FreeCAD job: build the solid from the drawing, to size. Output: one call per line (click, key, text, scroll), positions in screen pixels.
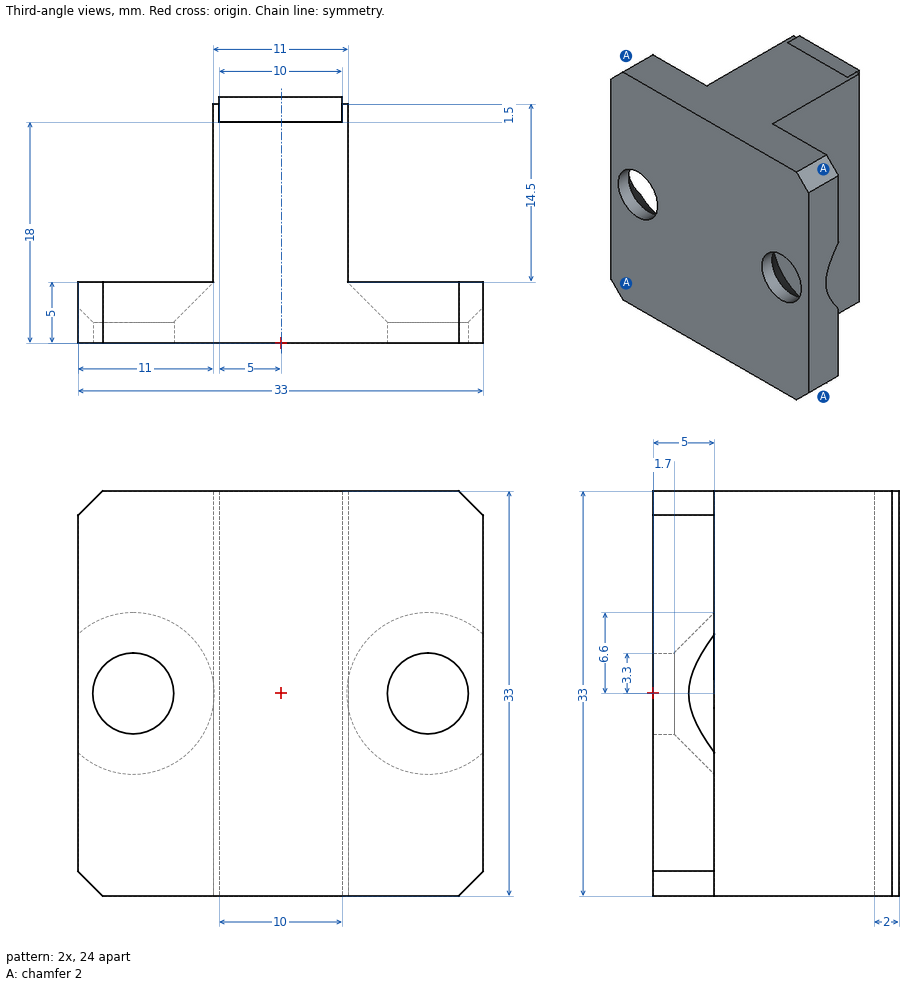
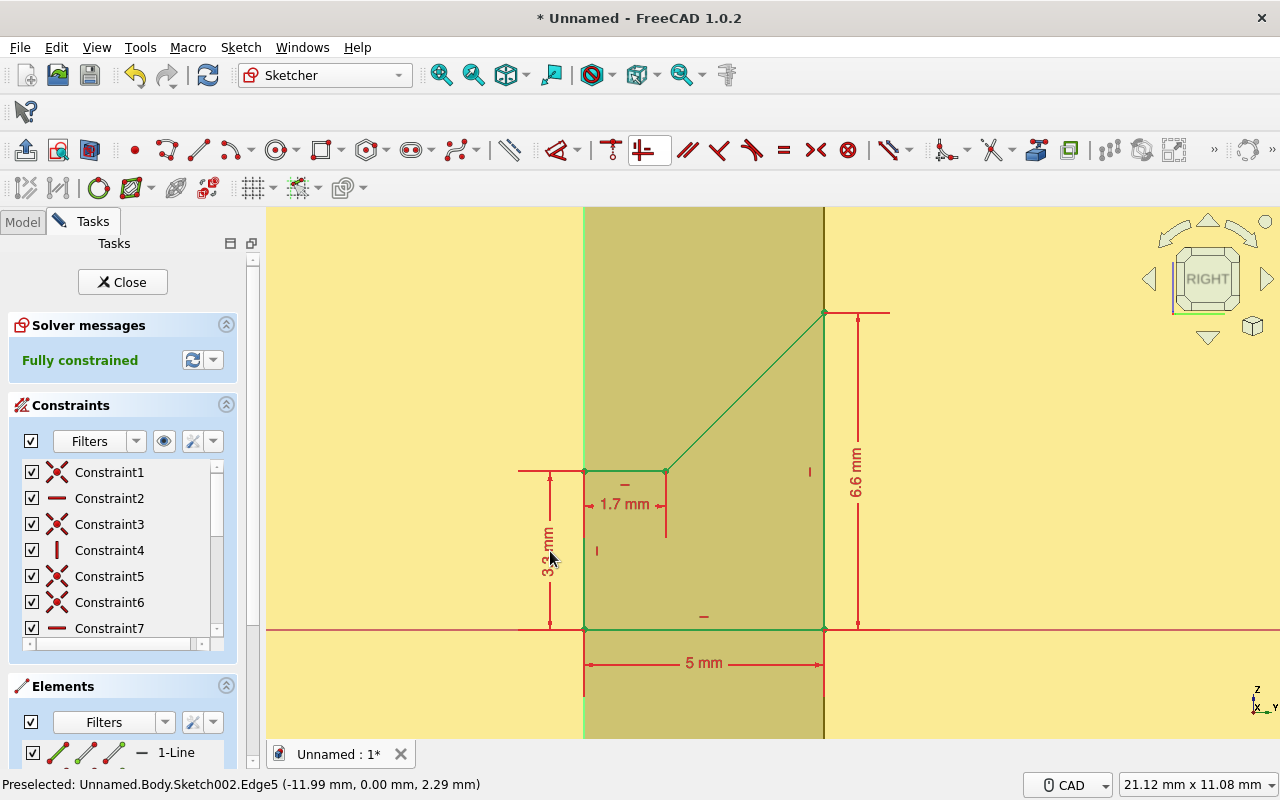
click(123, 282)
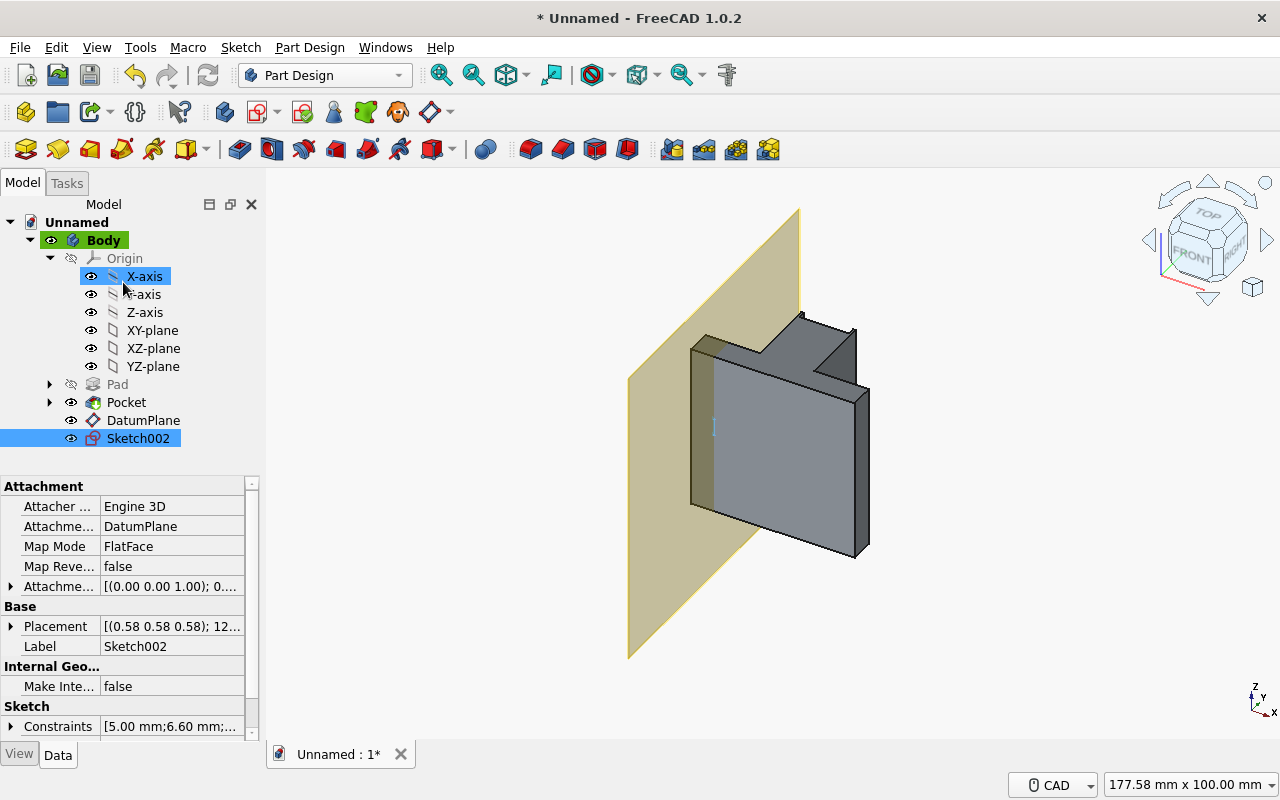
click(304, 150)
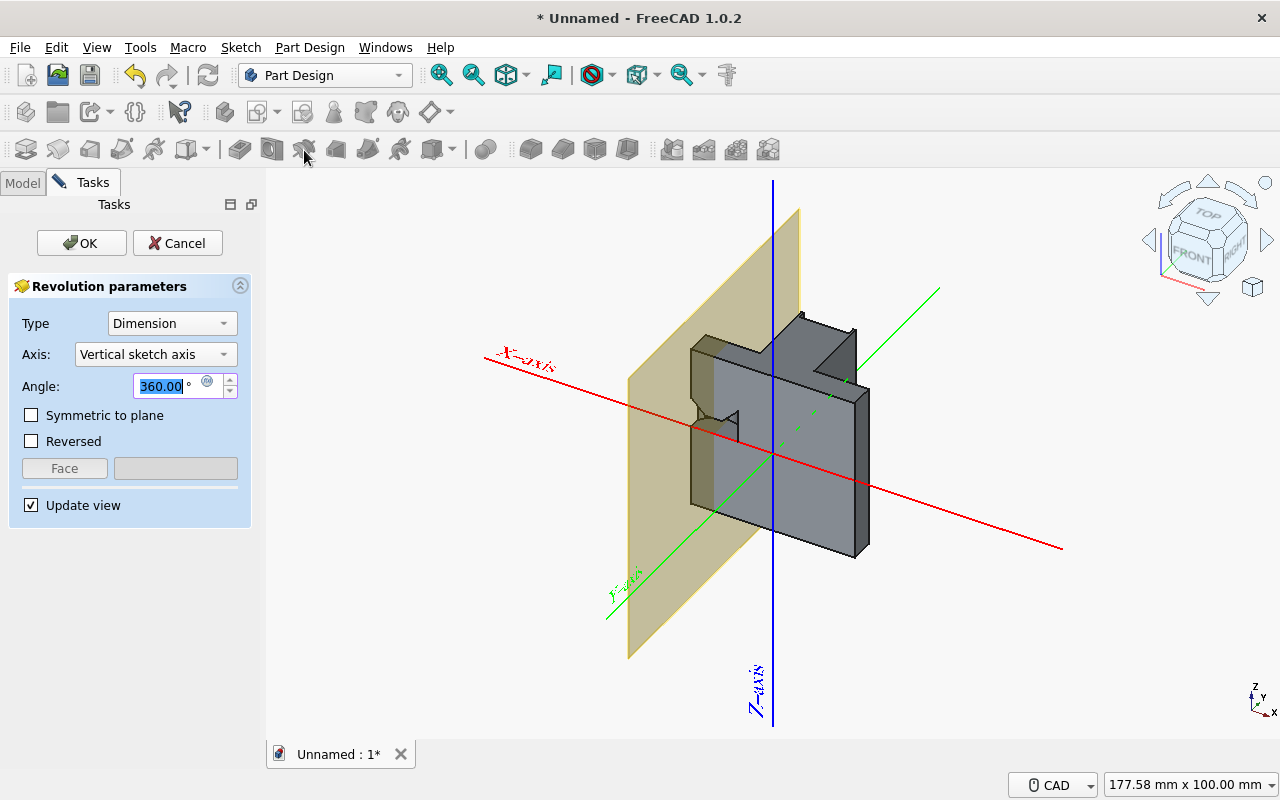
click(156, 354)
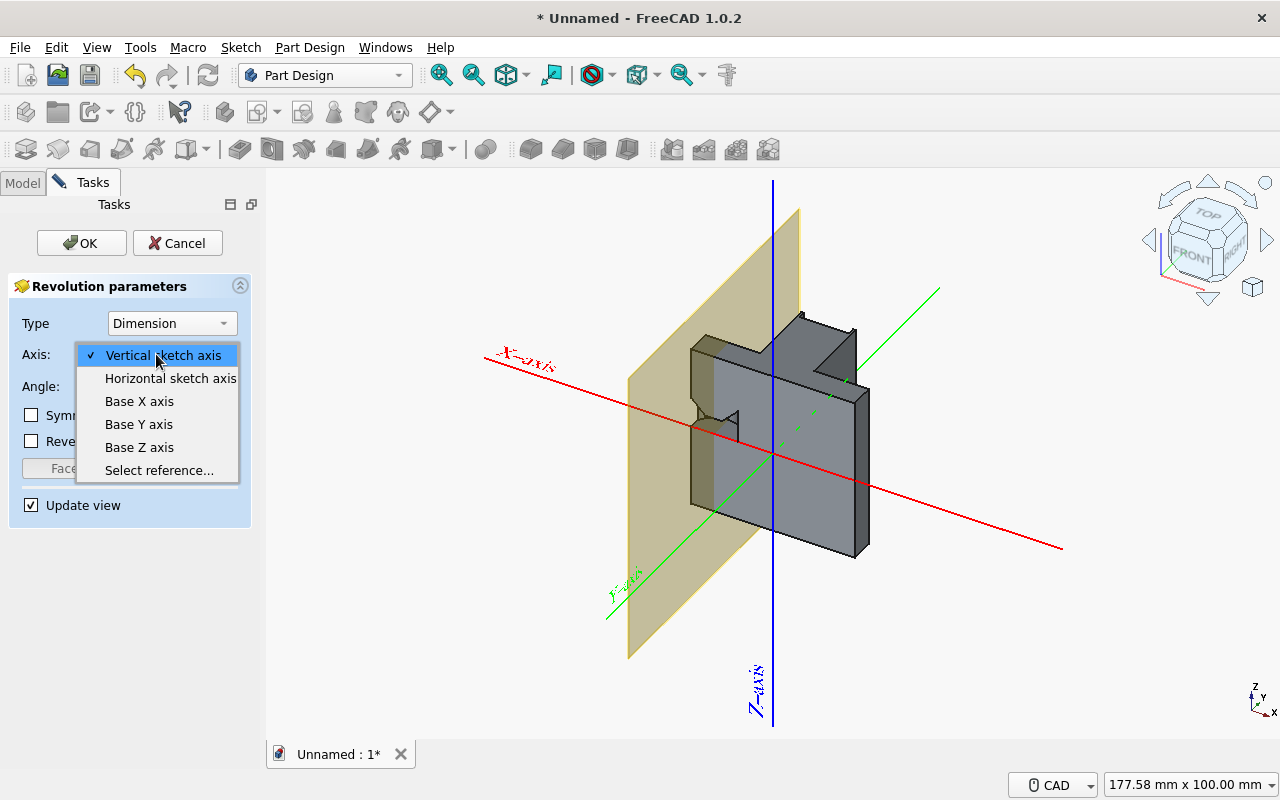
click(156, 378)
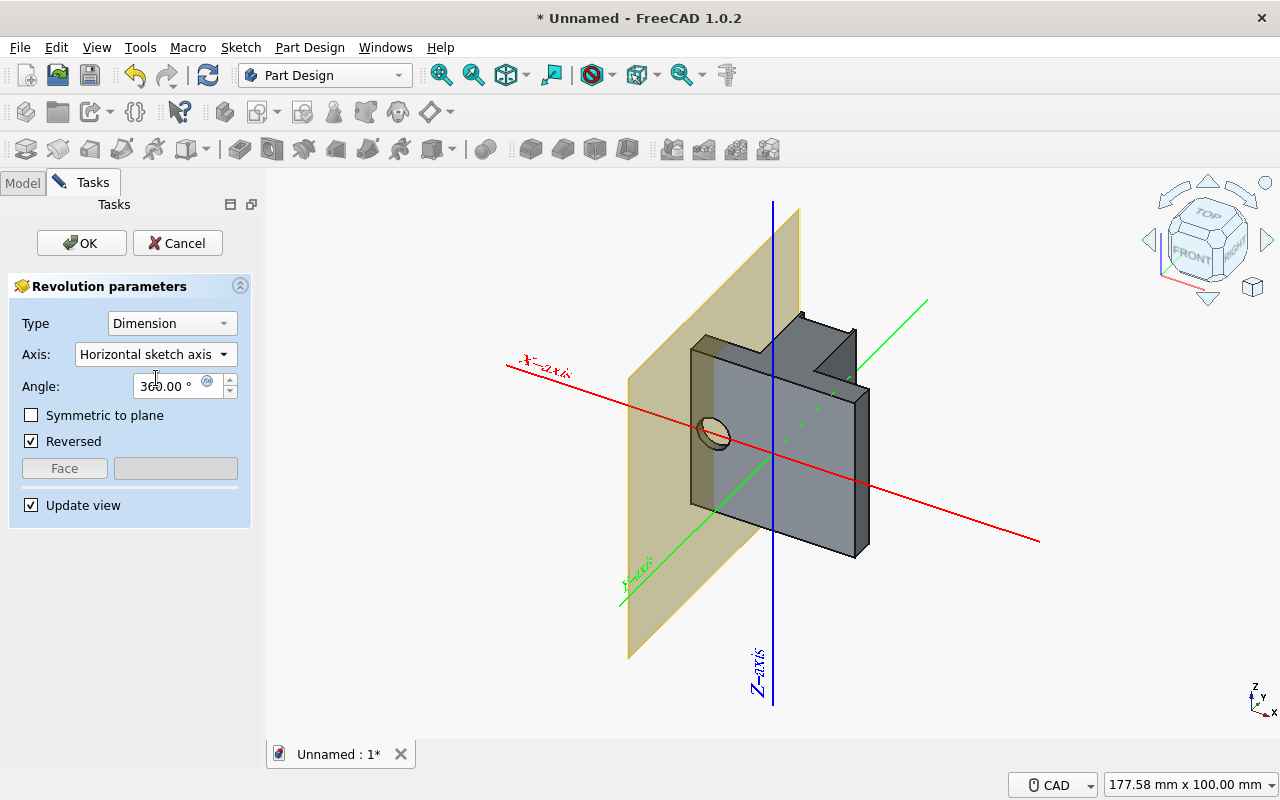
click(82, 243)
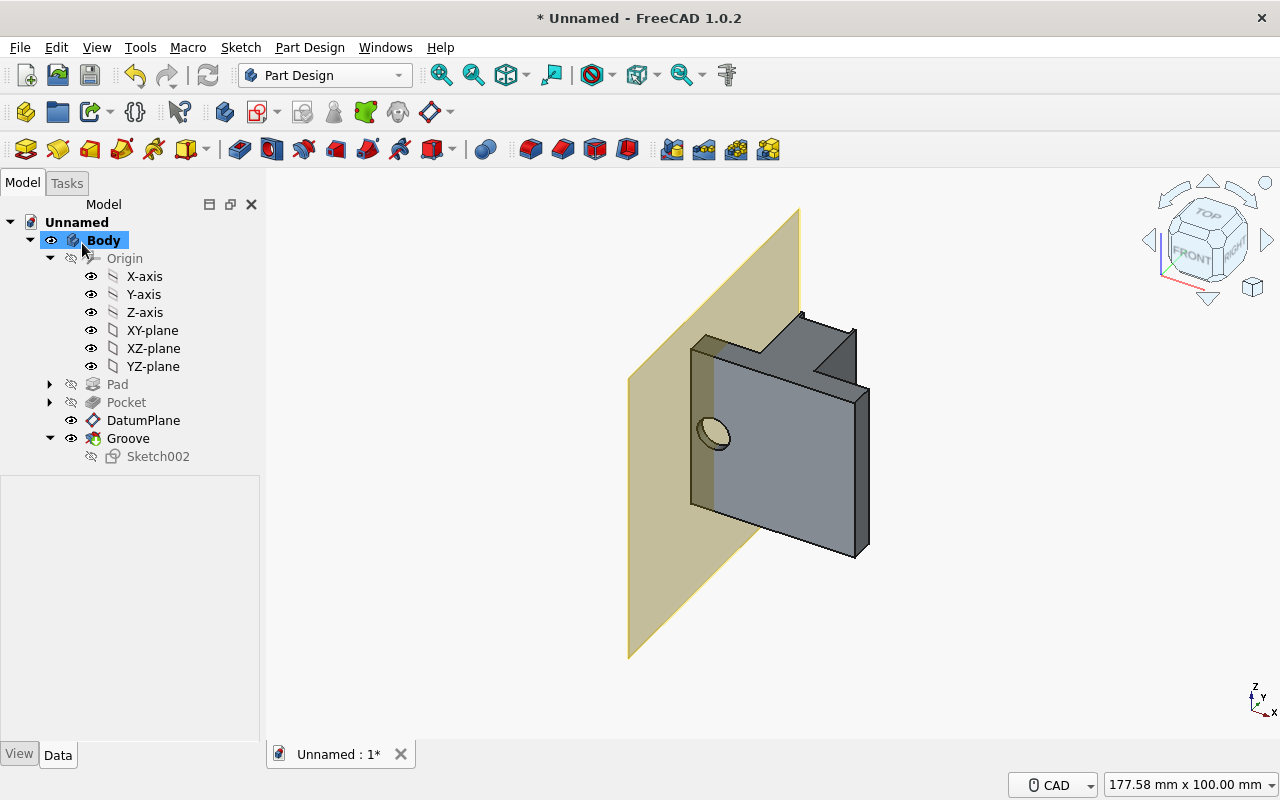
click(116, 420)
key(space)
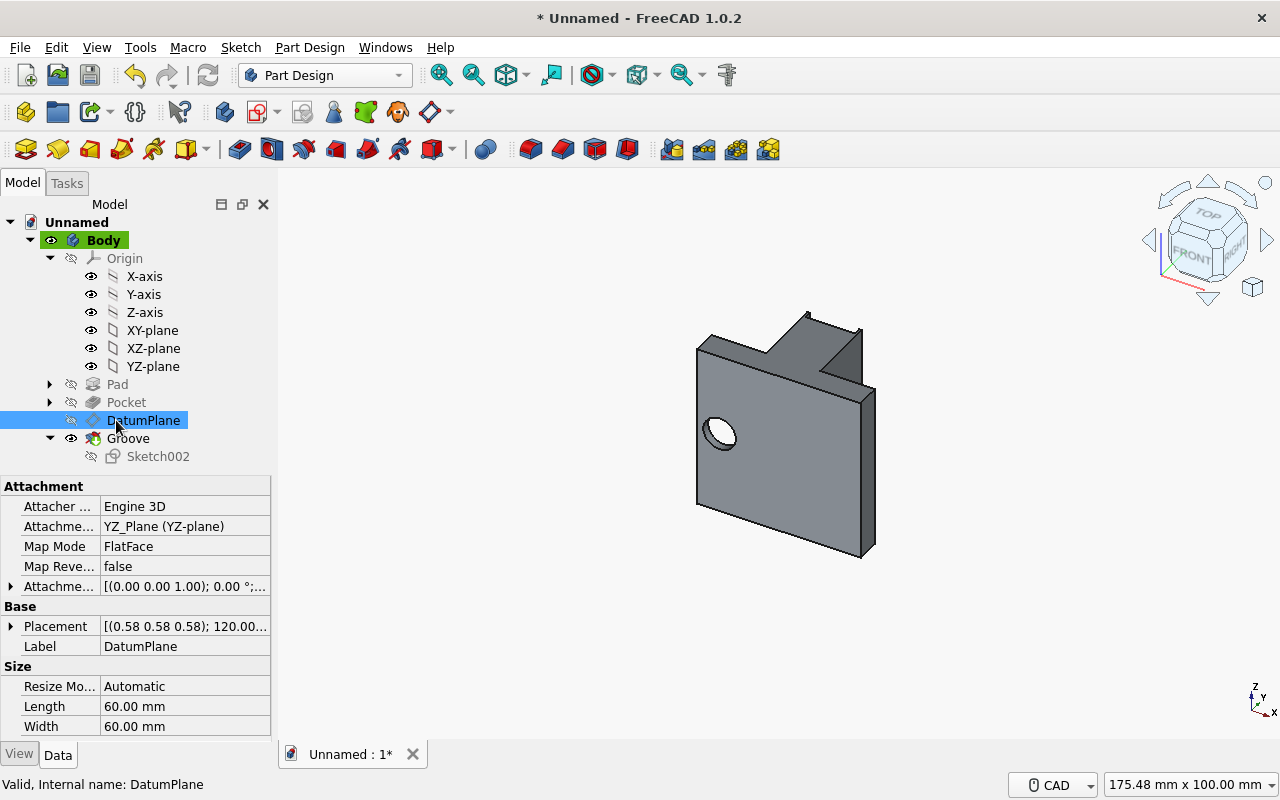
click(116, 438)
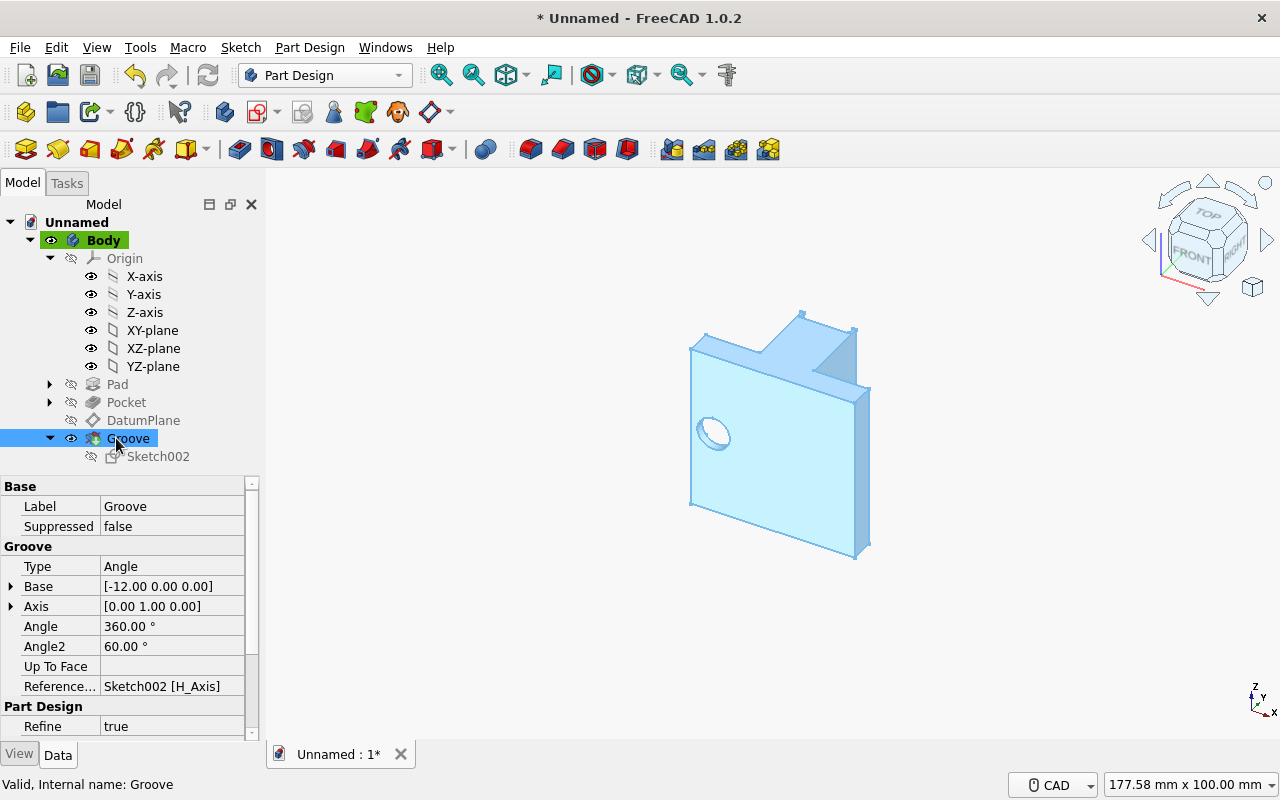
click(704, 150)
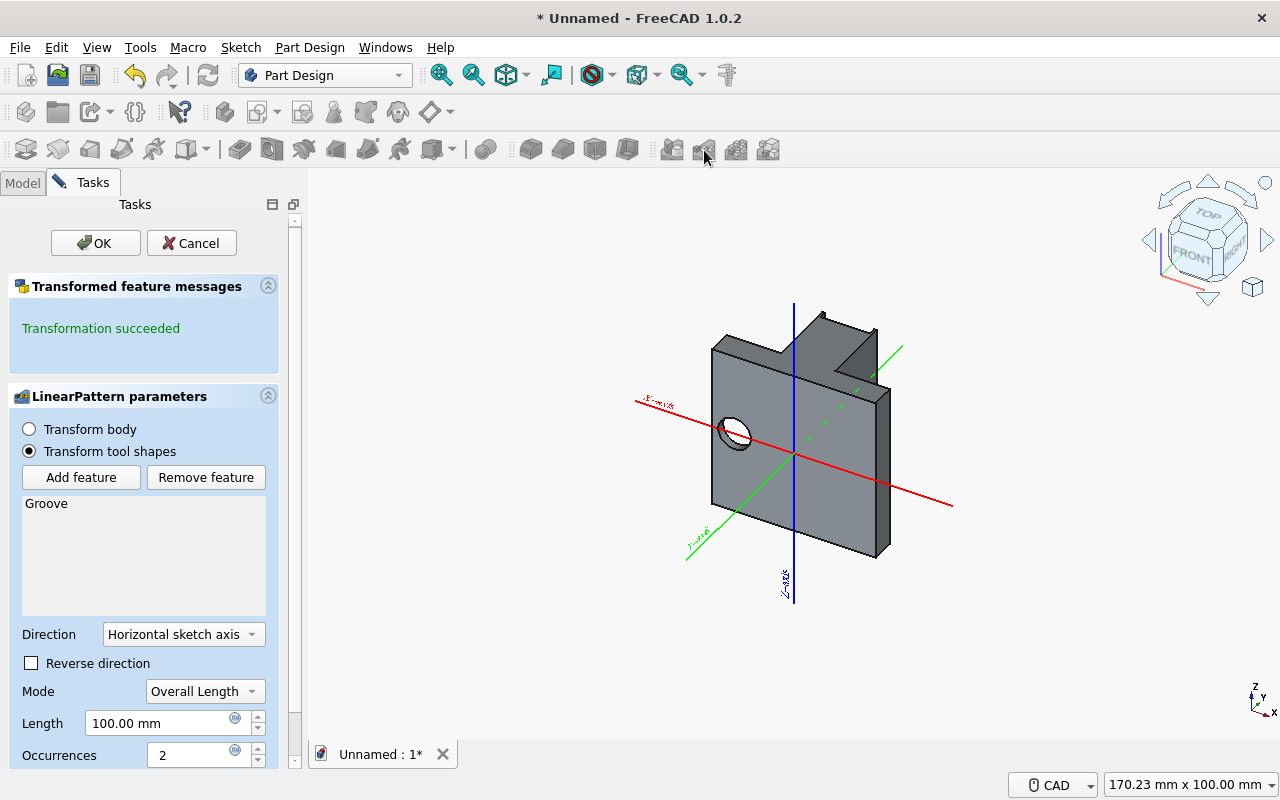
click(184, 634)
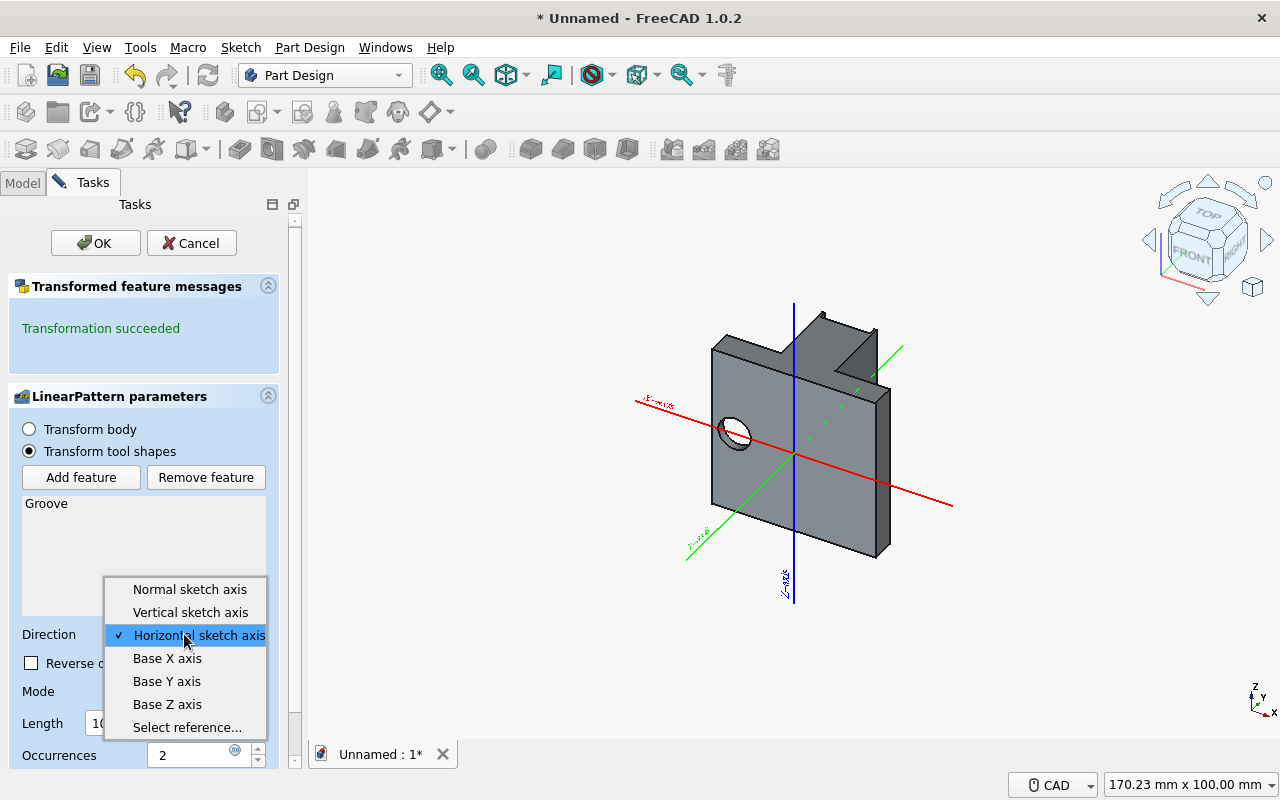
click(184, 658)